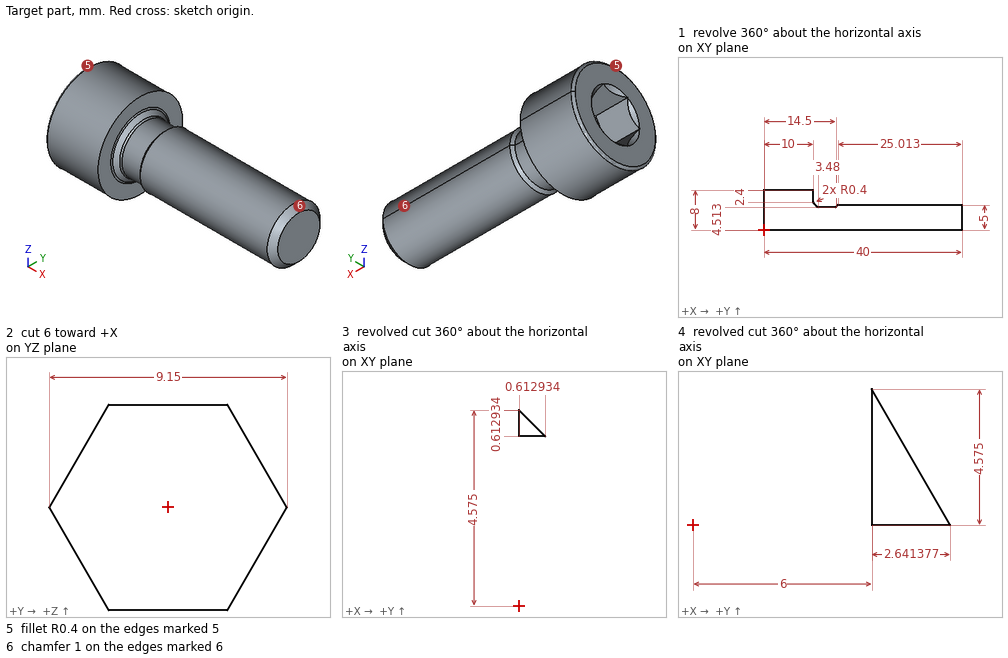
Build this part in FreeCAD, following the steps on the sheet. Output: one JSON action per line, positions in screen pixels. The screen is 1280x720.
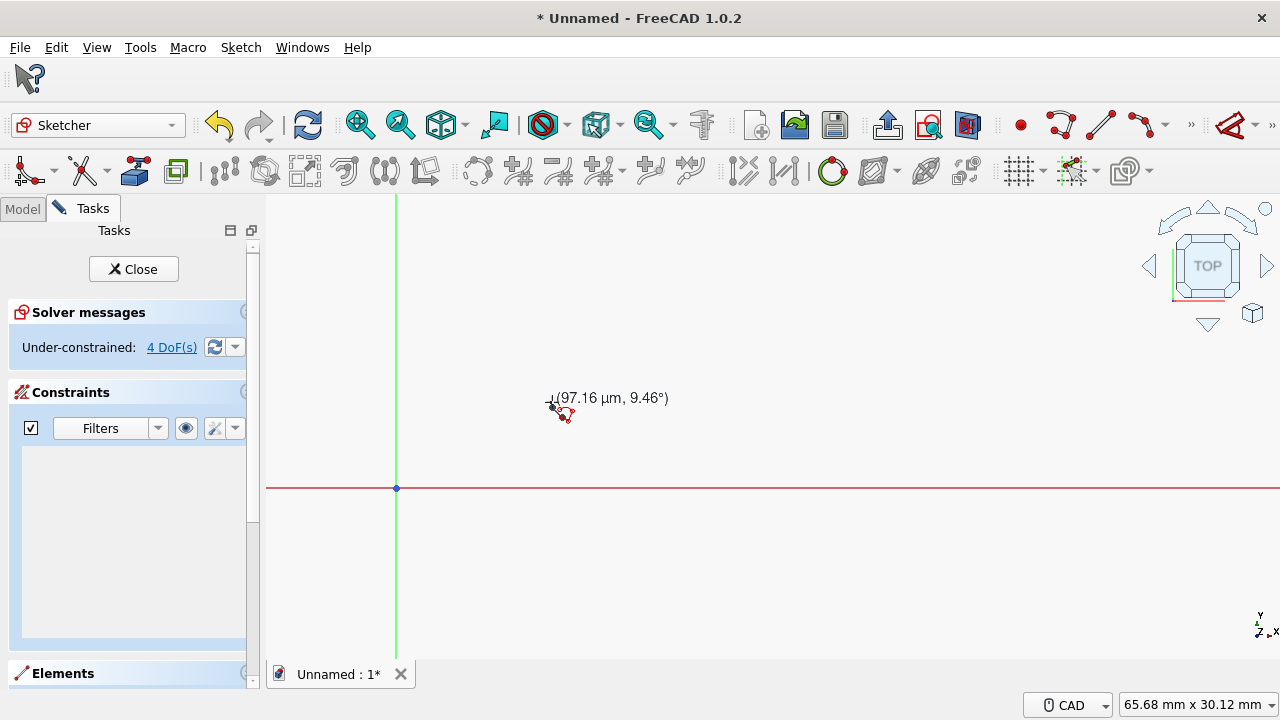
{"action": "left_click", "coordinate": [551, 365]}
{"action": "left_click", "coordinate": [396, 365]}
{"action": "left_click", "coordinate": [396, 488]}
{"action": "left_click", "coordinate": [1014, 479]}
{"action": "left_click", "coordinate": [1014, 411]}
{"action": "left_click", "coordinate": [628, 411]}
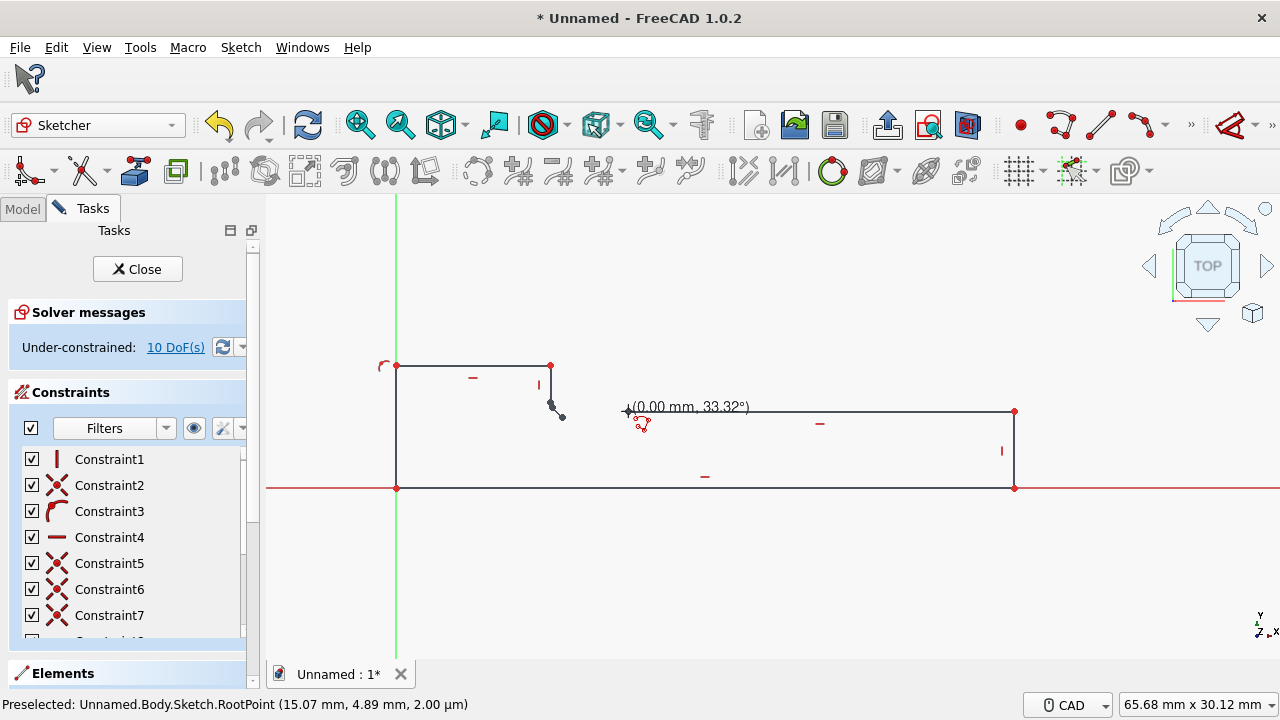
{"action": "scroll", "coordinate": [620, 419], "scroll_direction": "up", "scroll_amount": 3}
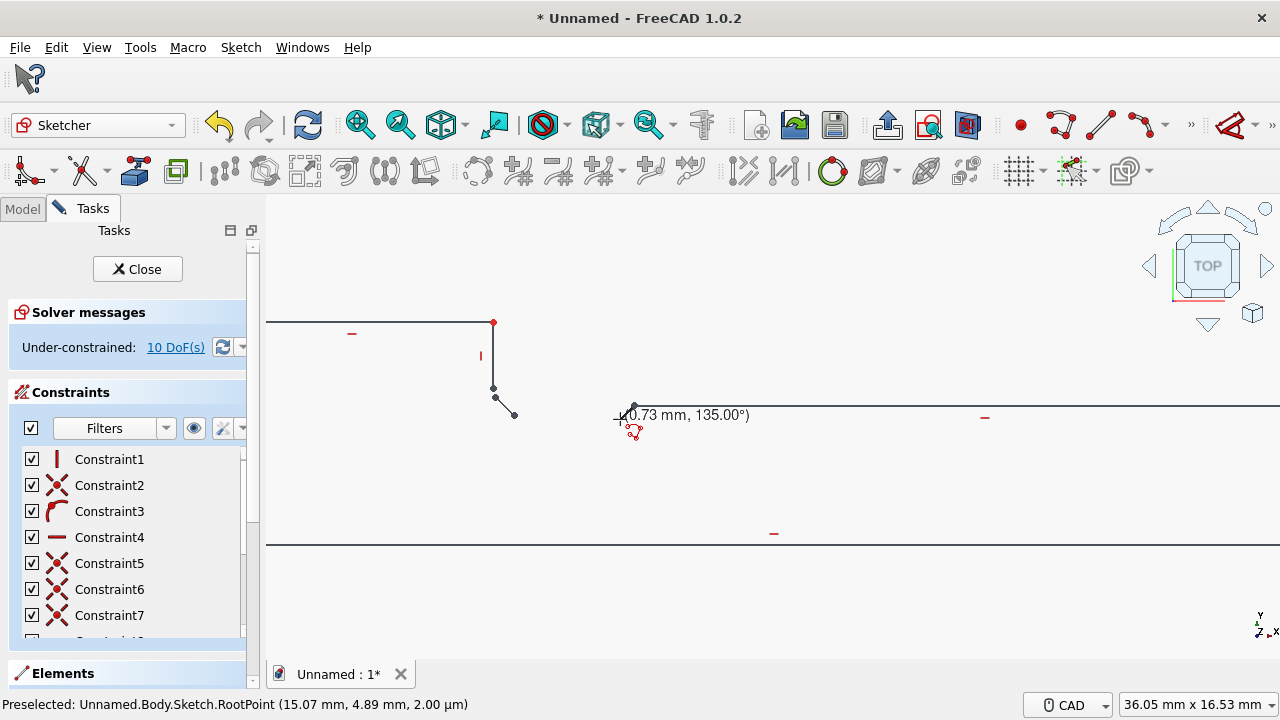
{"action": "left_click", "coordinate": [620, 418]}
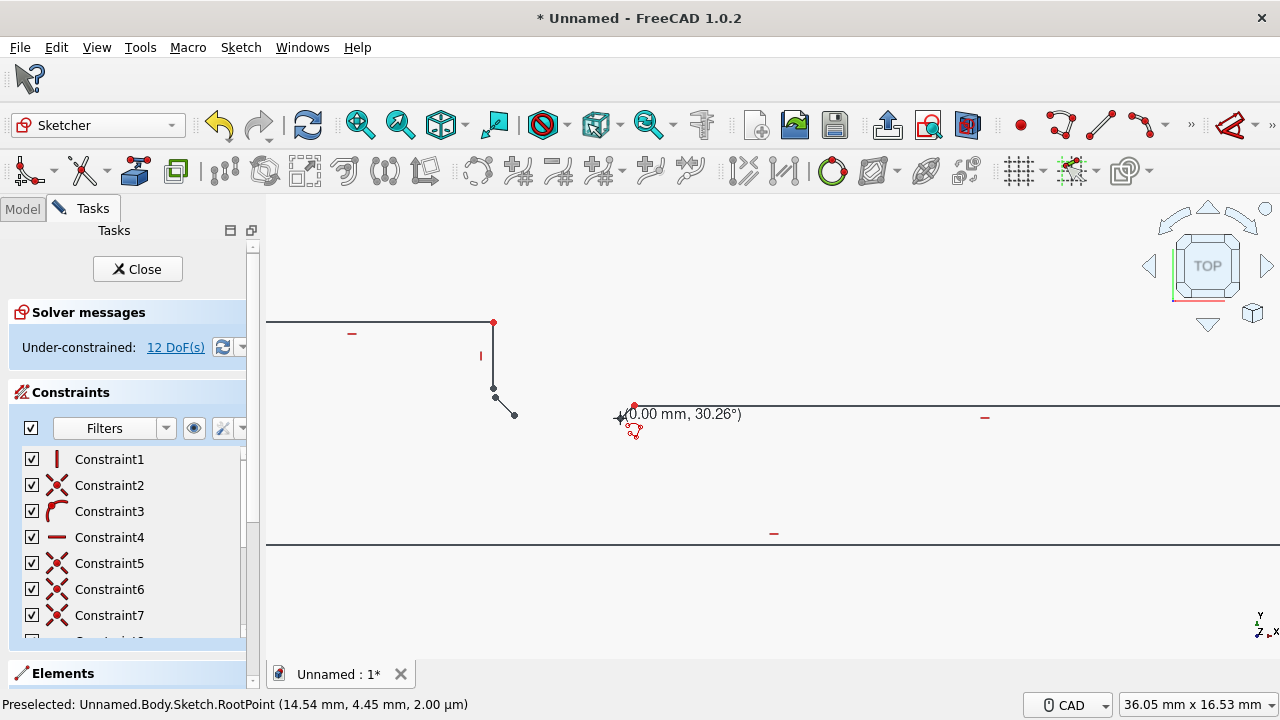
{"action": "scroll", "coordinate": [522, 418], "scroll_direction": "up", "scroll_amount": 3}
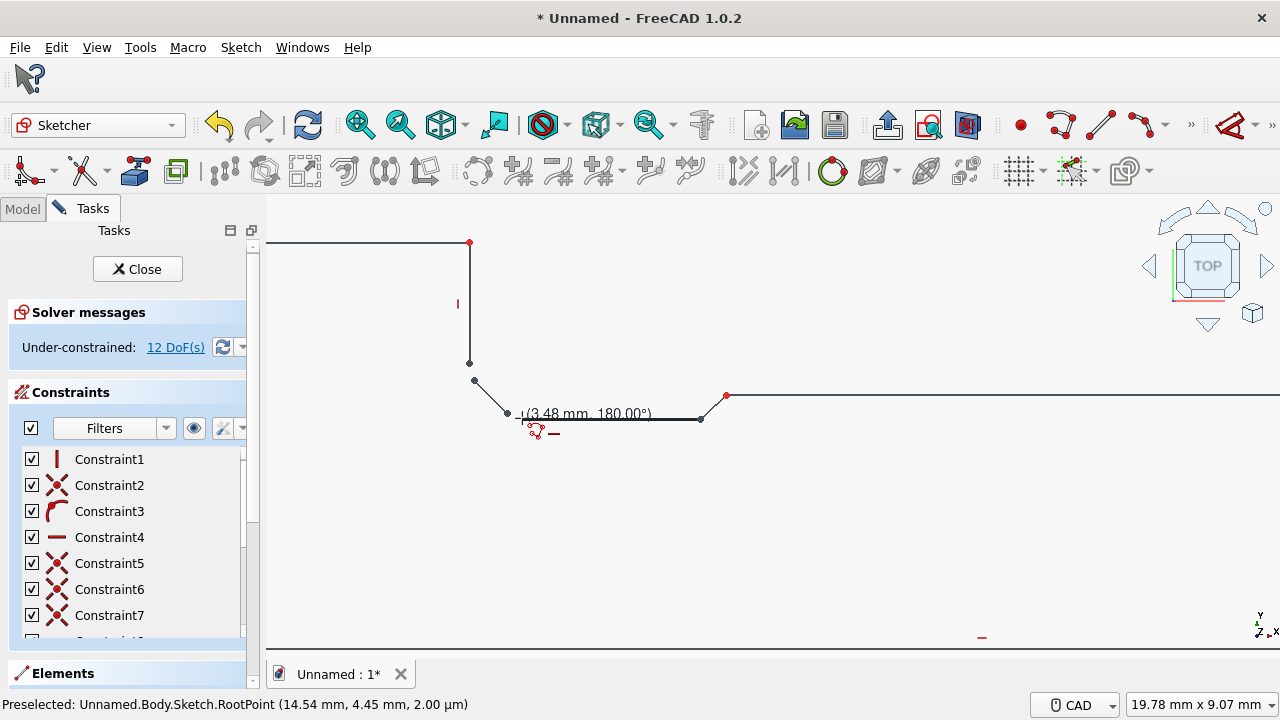
{"action": "left_click", "coordinate": [522, 418]}
{"action": "right_click", "coordinate": [522, 418]}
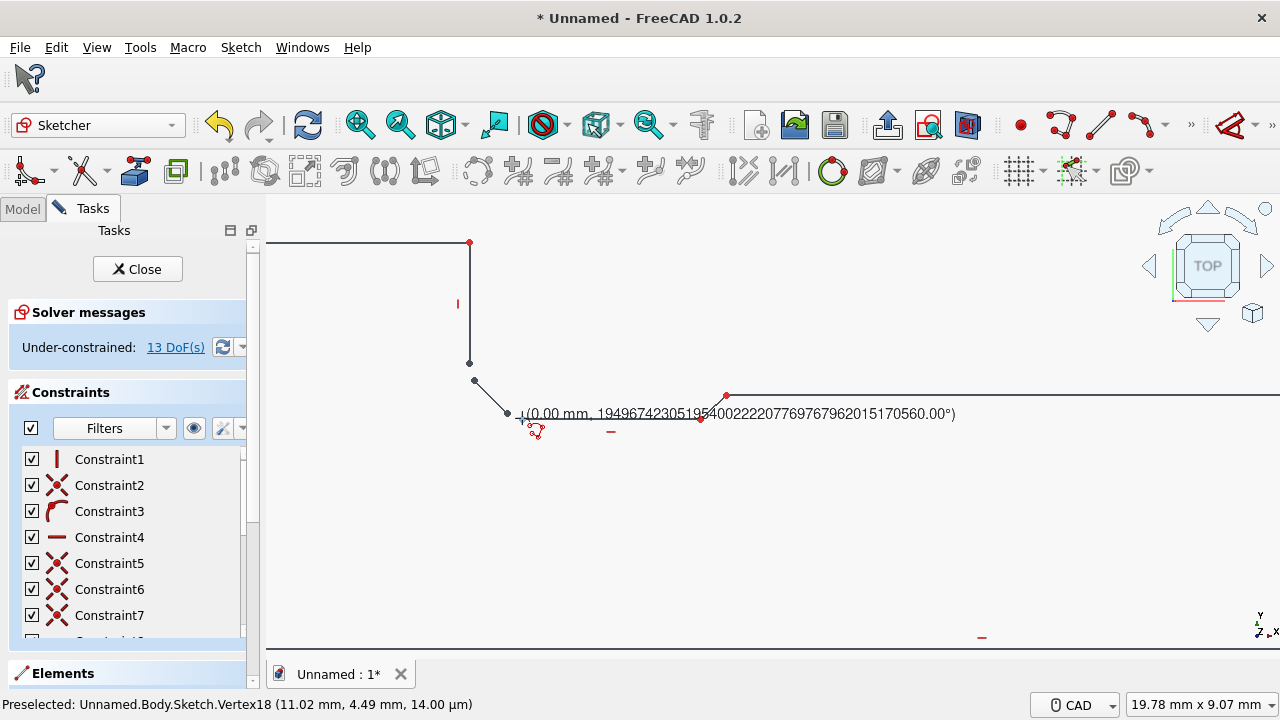
{"action": "left_click", "coordinate": [1142, 126]}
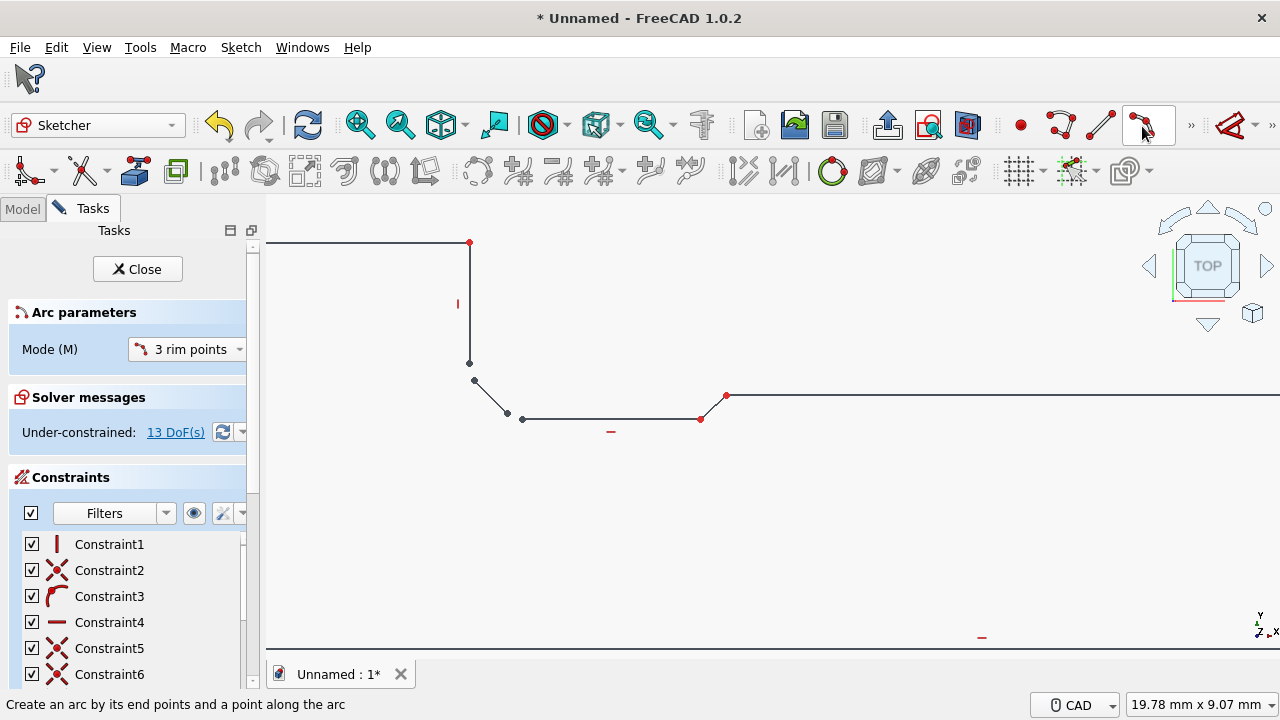
{"action": "left_click", "coordinate": [474, 381]}
{"action": "left_click", "coordinate": [470, 363]}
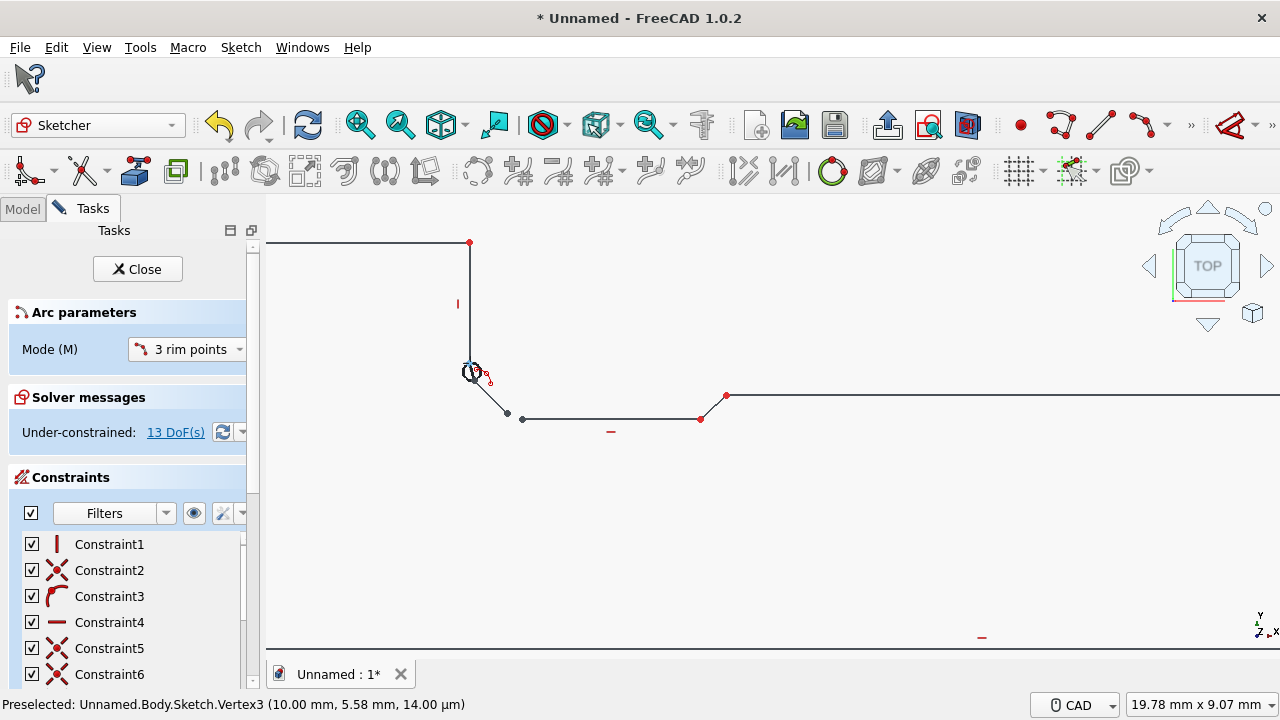
{"action": "scroll", "coordinate": [471, 370], "scroll_direction": "up", "scroll_amount": 13}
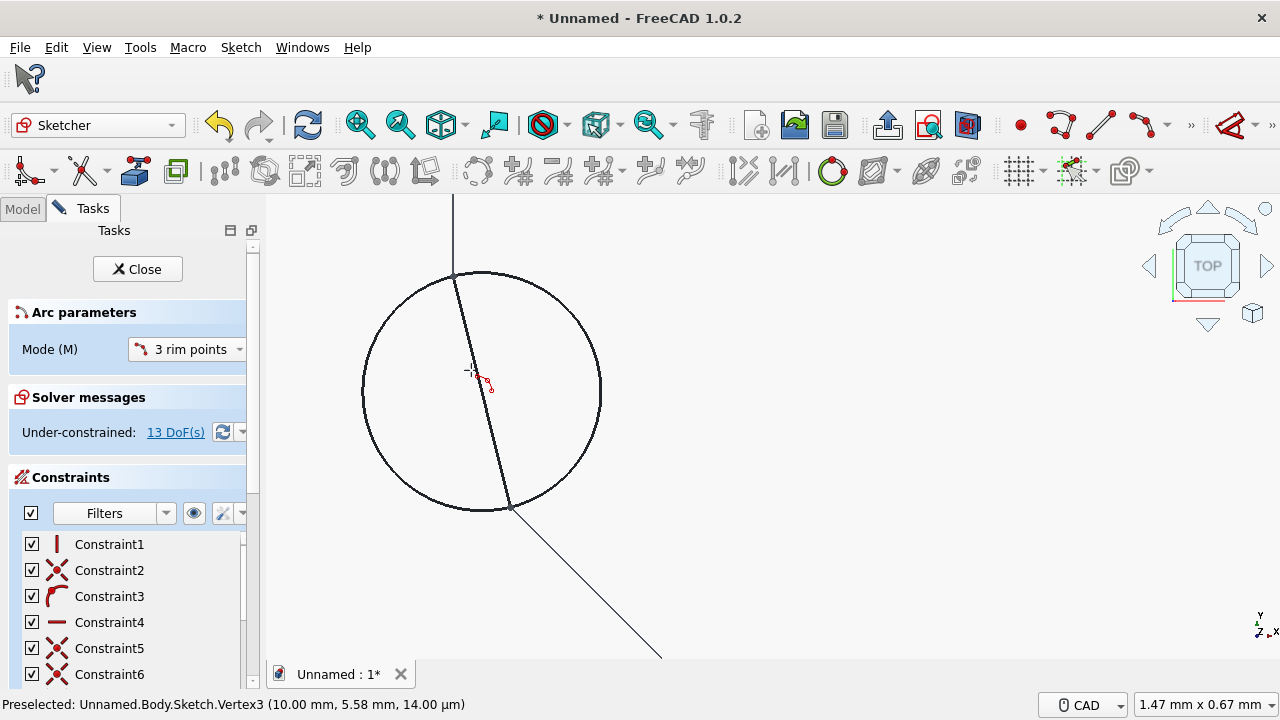
{"action": "left_click", "coordinate": [470, 360]}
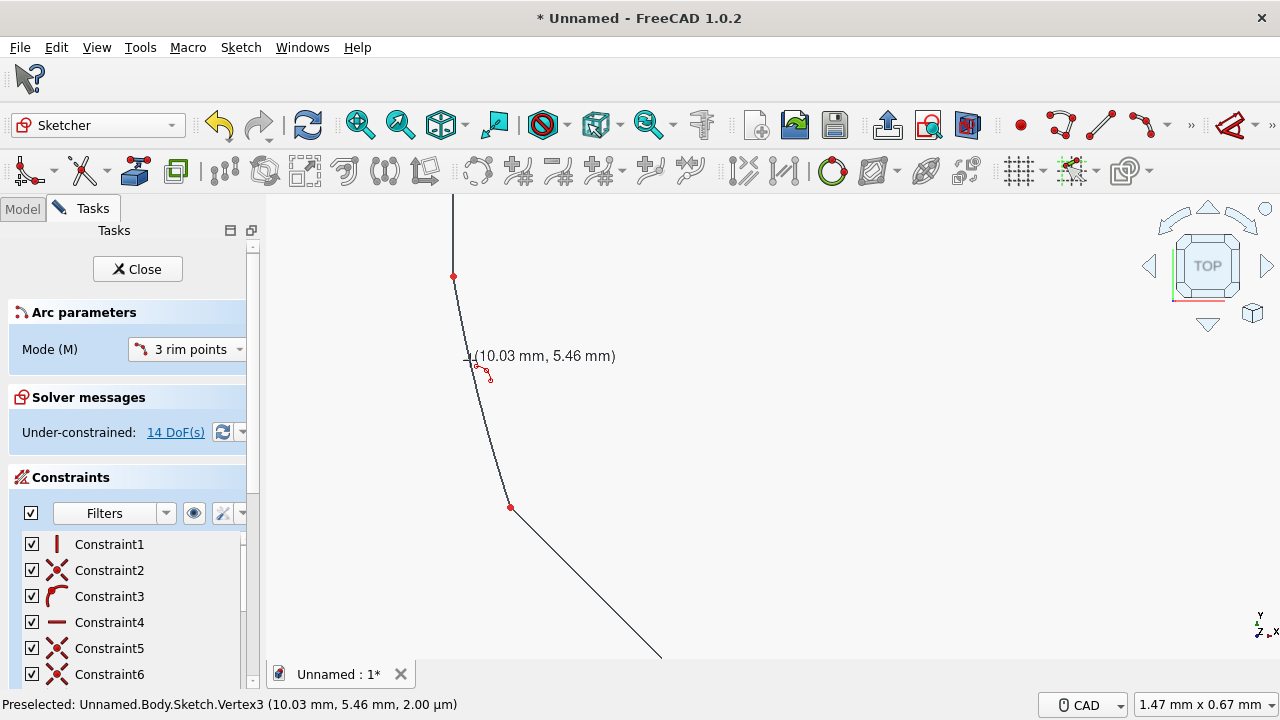
{"action": "scroll", "coordinate": [518, 400], "scroll_direction": "down", "scroll_amount": 18}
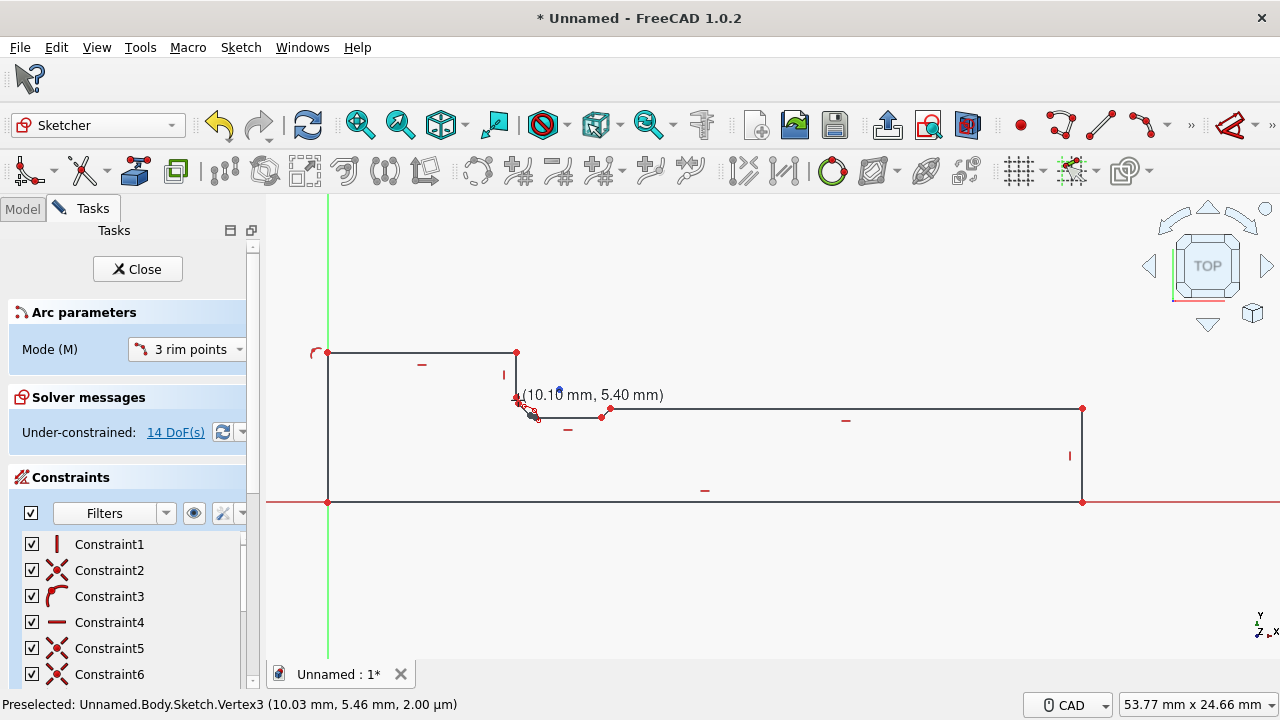
{"action": "scroll", "coordinate": [536, 417], "scroll_direction": "up", "scroll_amount": 5}